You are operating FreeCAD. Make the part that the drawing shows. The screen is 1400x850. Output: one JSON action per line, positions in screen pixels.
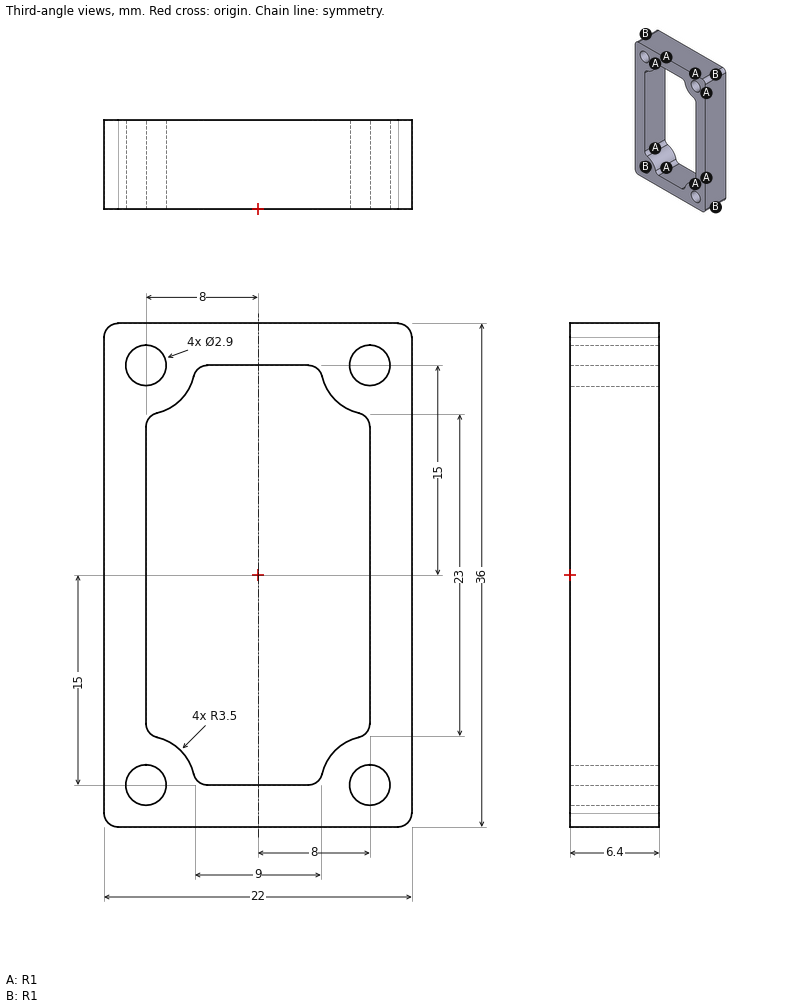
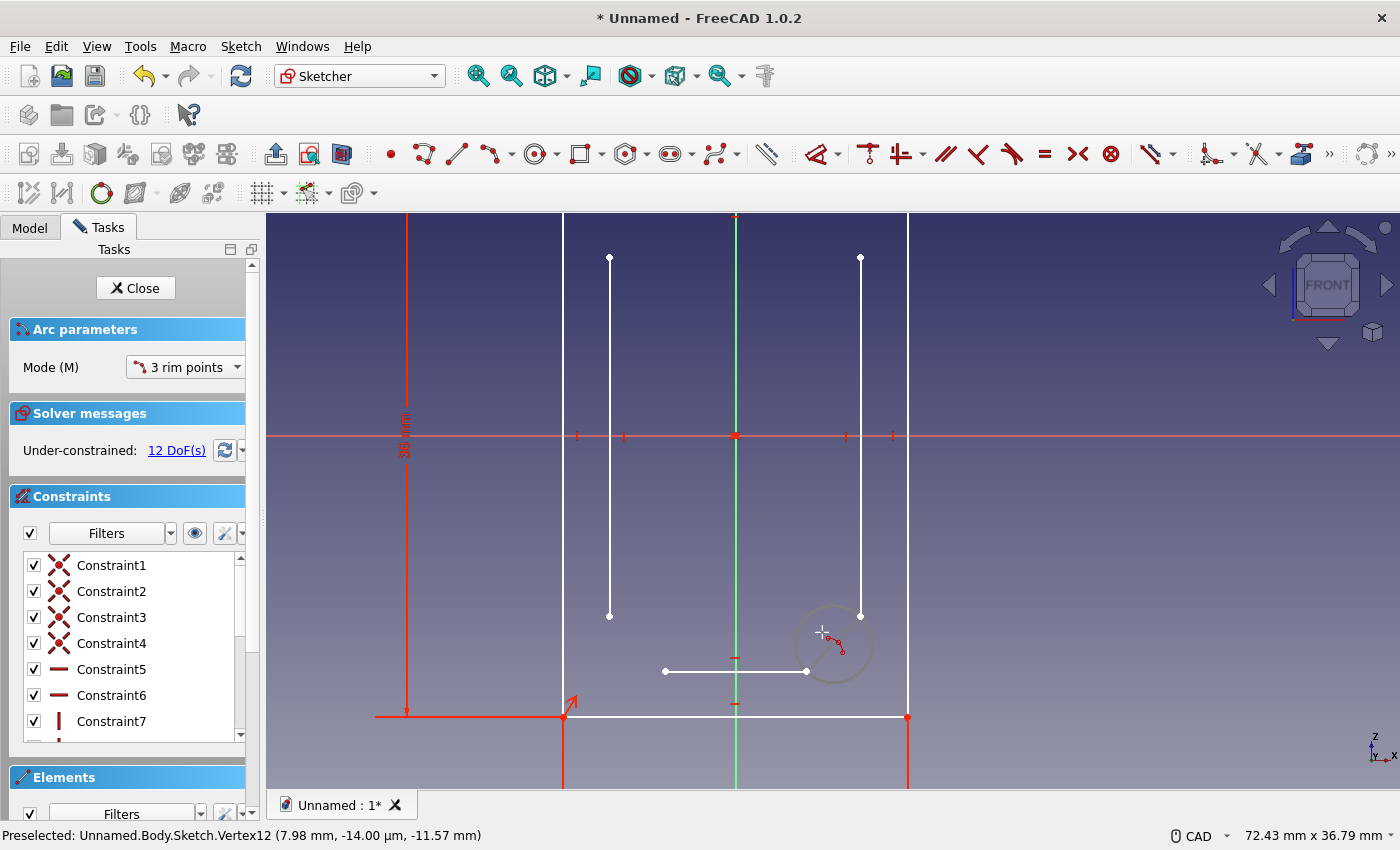
{"action": "left_click", "coordinate": [822, 632]}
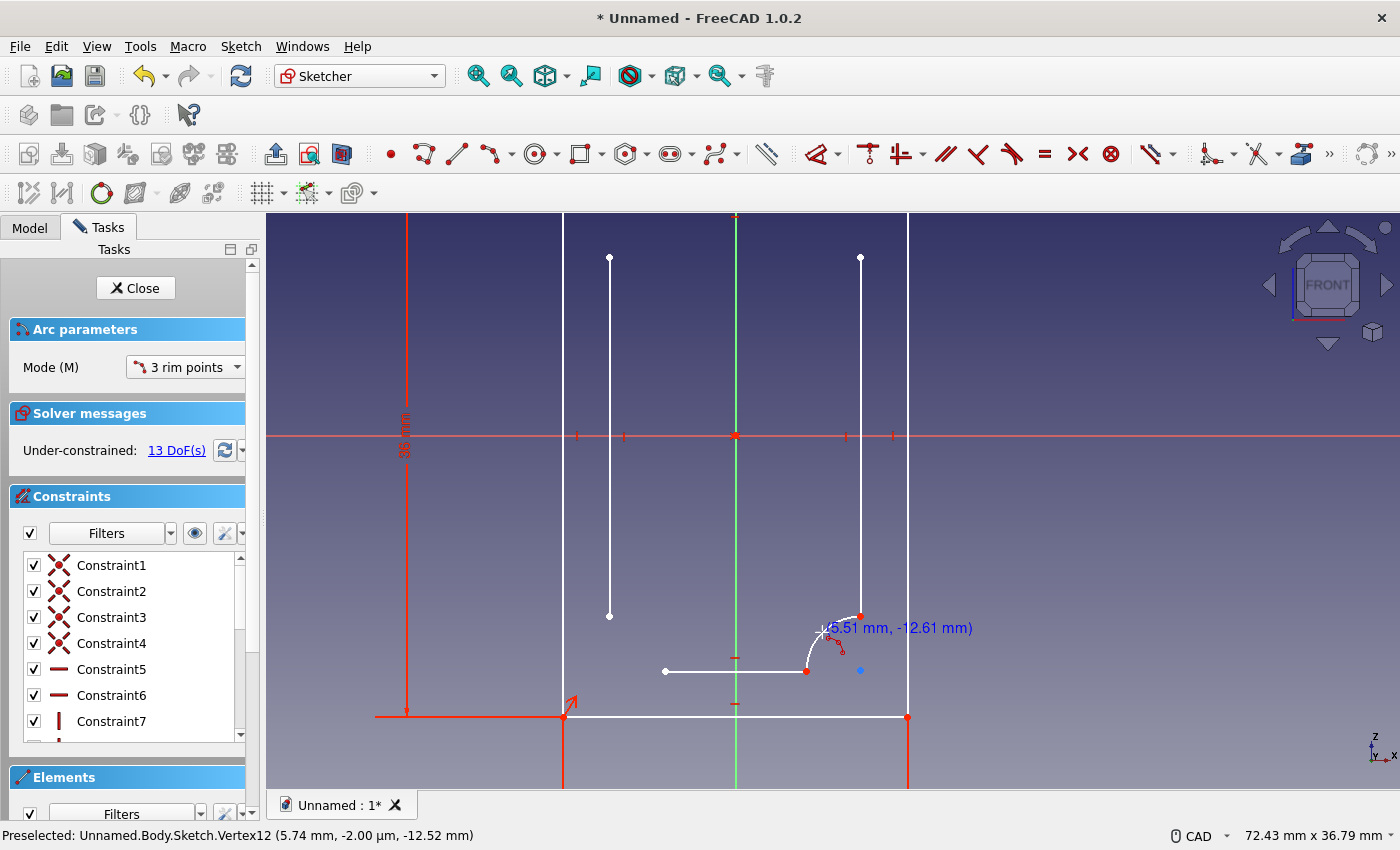
{"action": "left_click", "coordinate": [861, 257]}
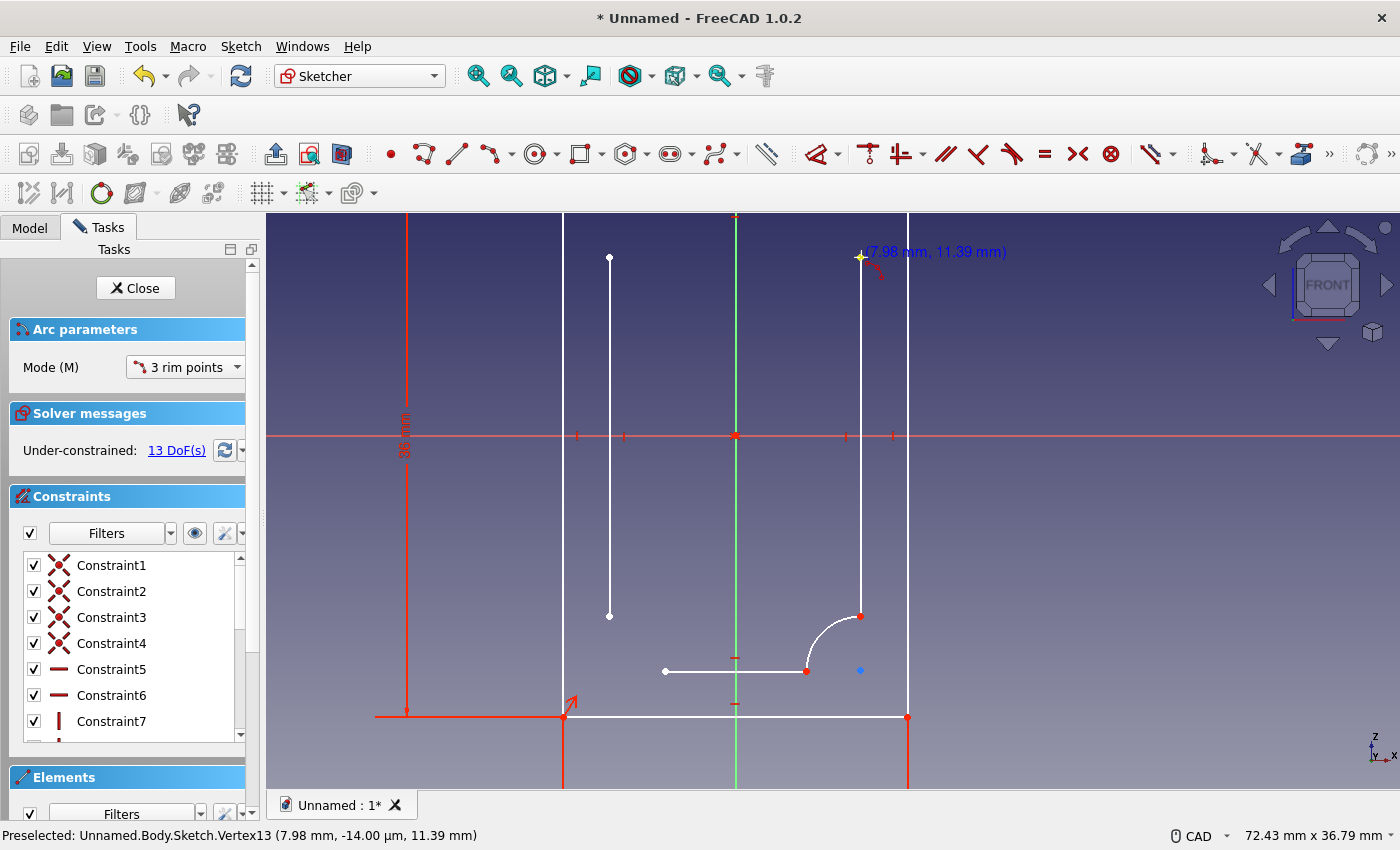
{"action": "scroll", "coordinate": [823, 634], "scroll_direction": "down", "scroll_amount": 2}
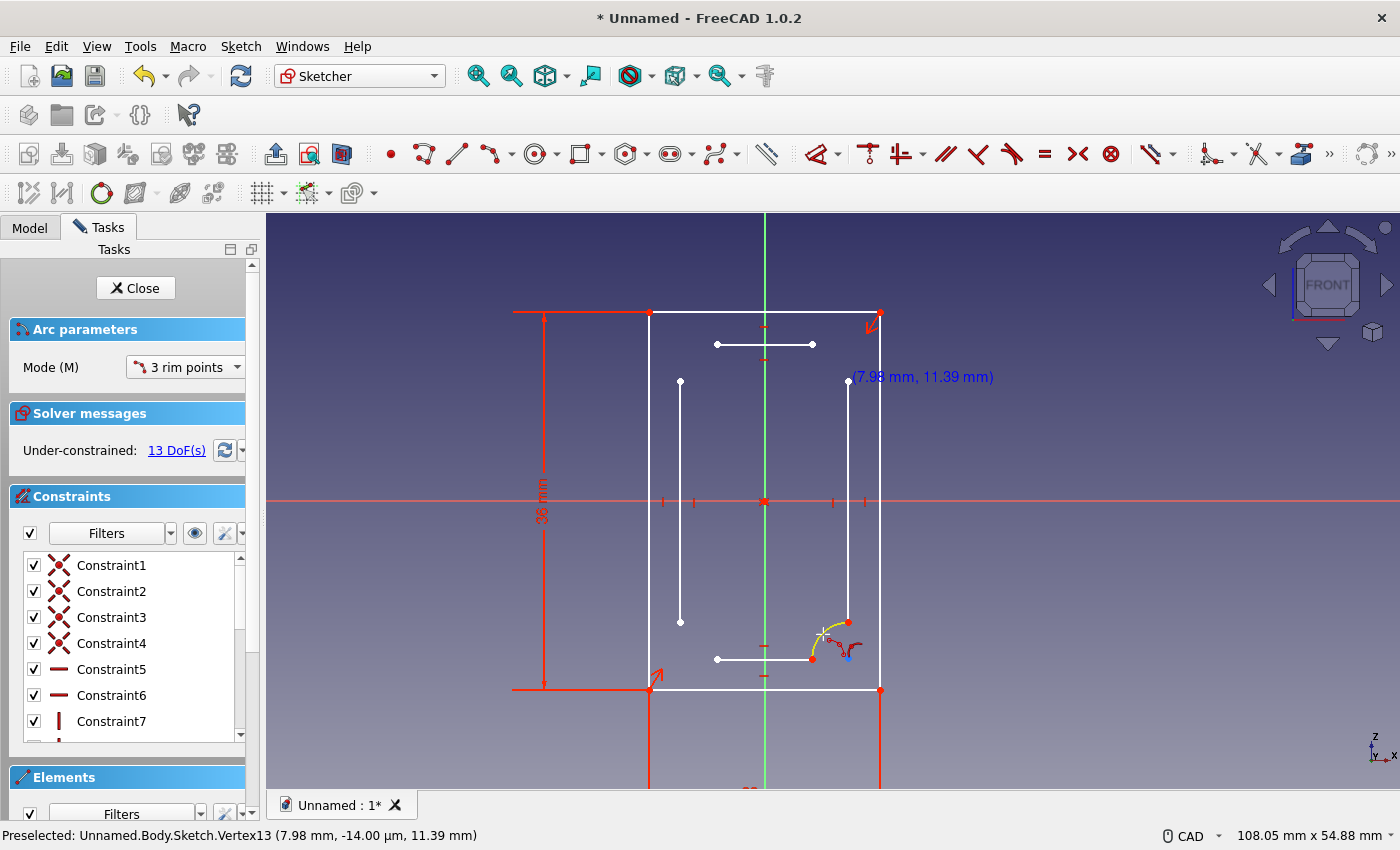
{"action": "left_click", "coordinate": [812, 345]}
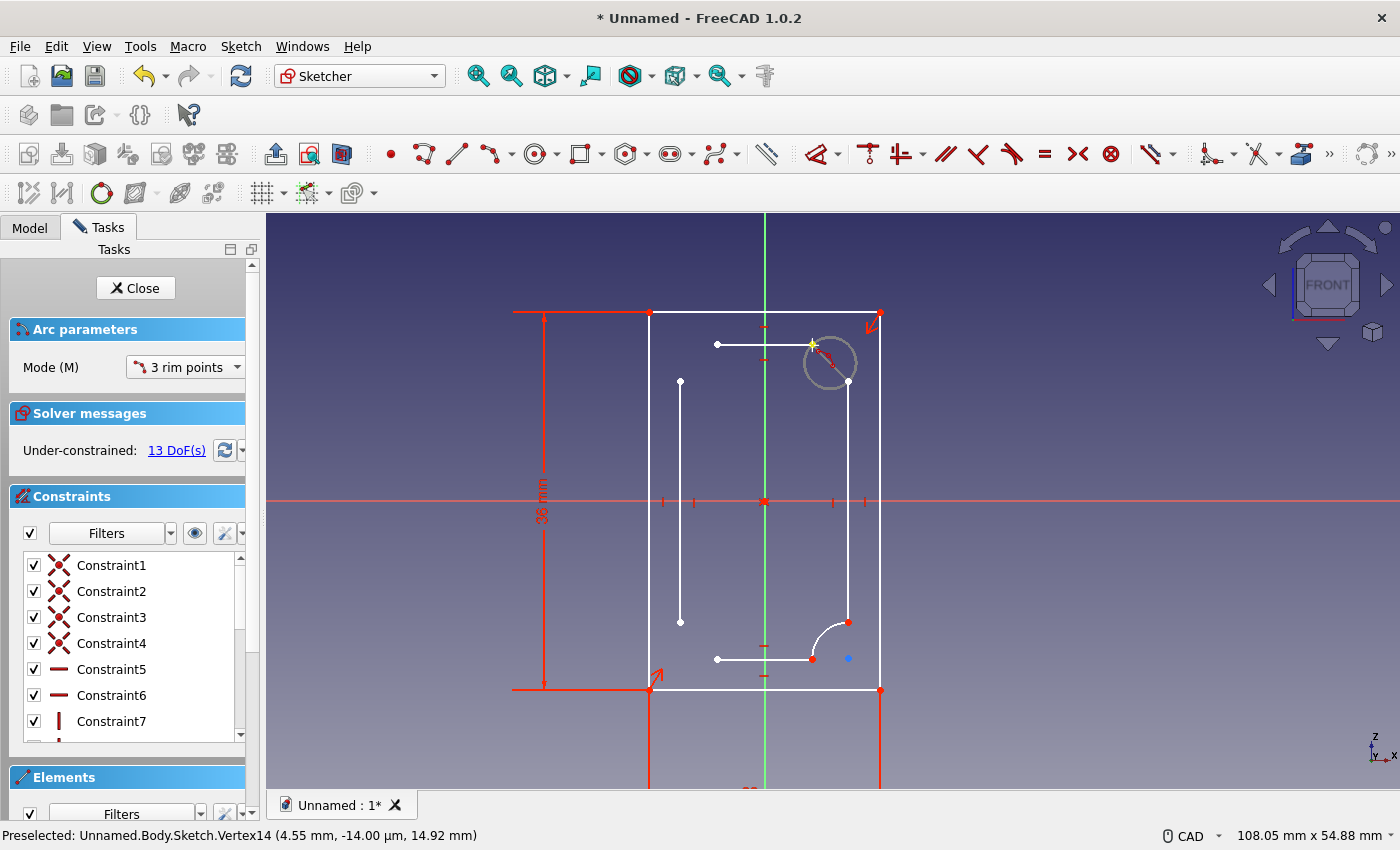
{"action": "scroll", "coordinate": [823, 370], "scroll_direction": "up", "scroll_amount": 2}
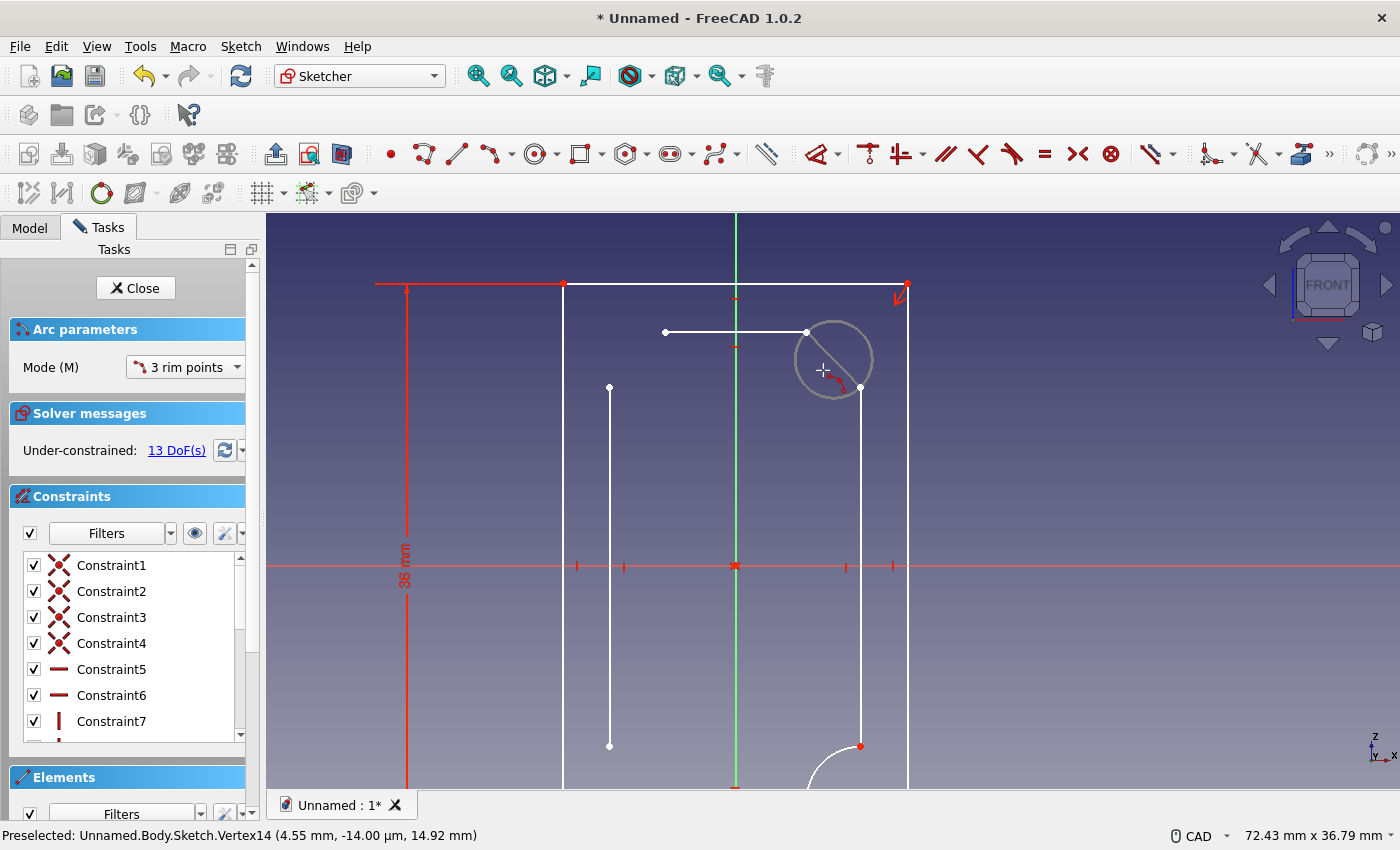
{"action": "left_click", "coordinate": [822, 370]}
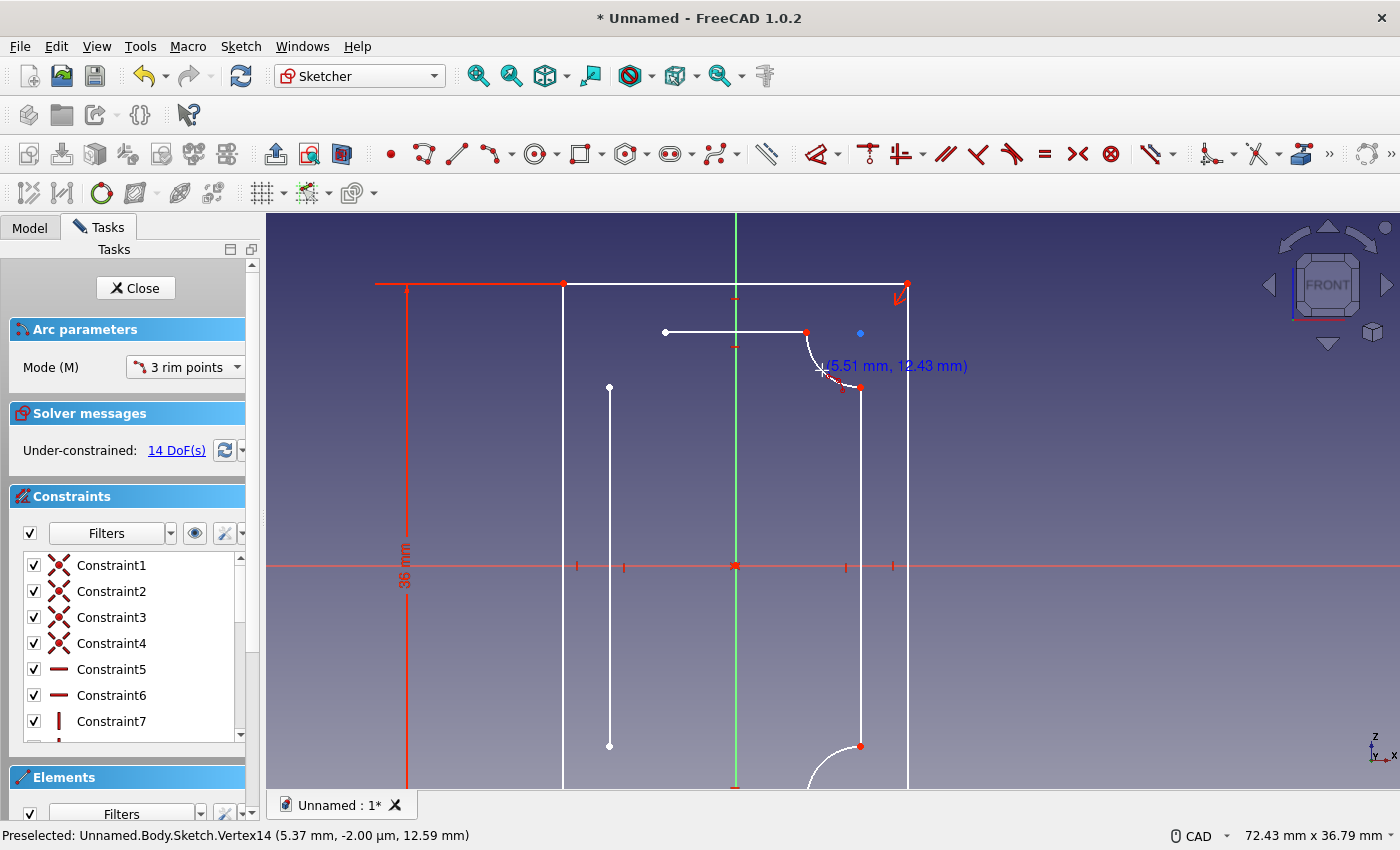
{"action": "left_click", "coordinate": [665, 332]}
{"action": "left_click", "coordinate": [610, 387]}
{"action": "left_click", "coordinate": [649, 370]}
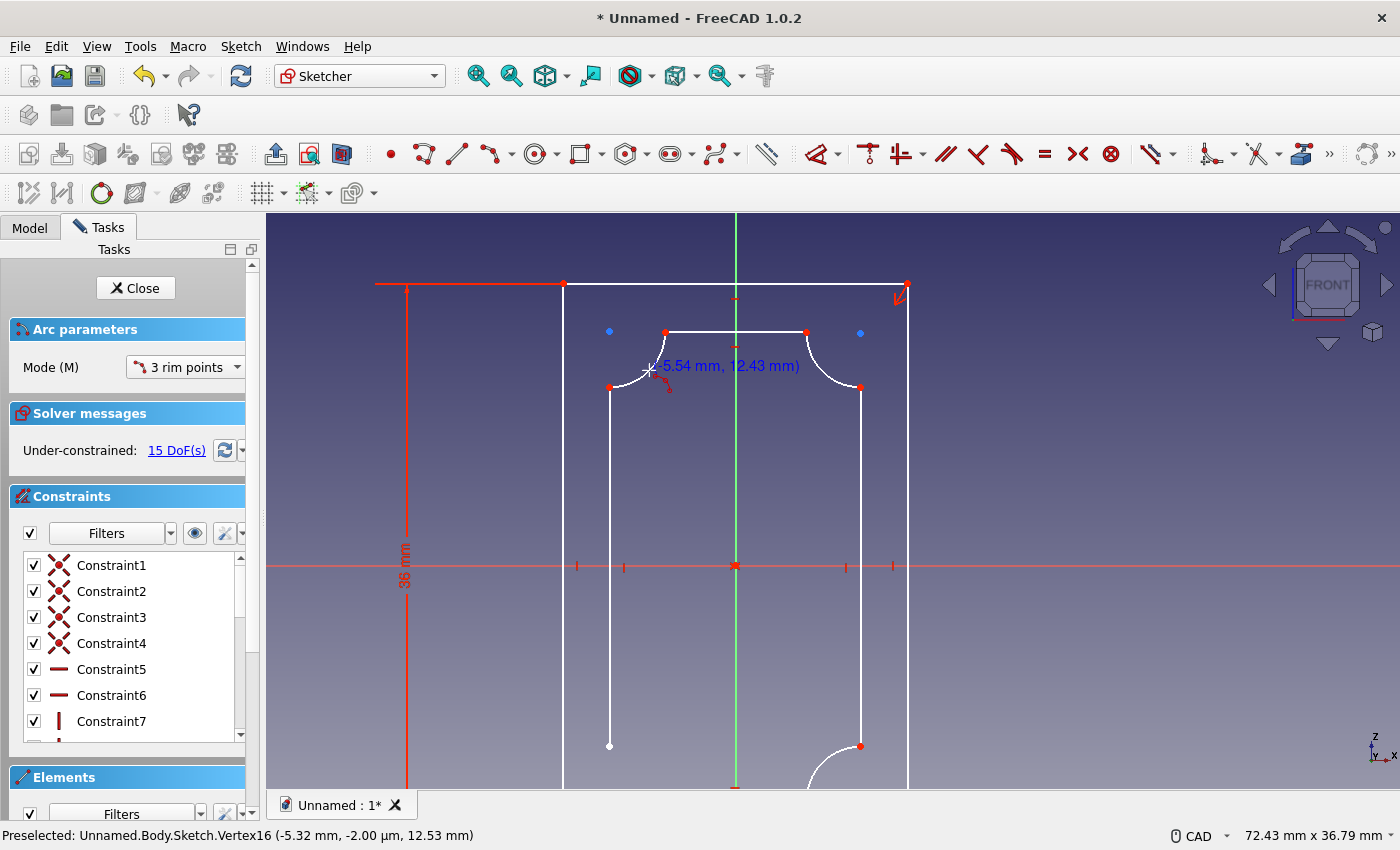
{"action": "left_click", "coordinate": [610, 747]}